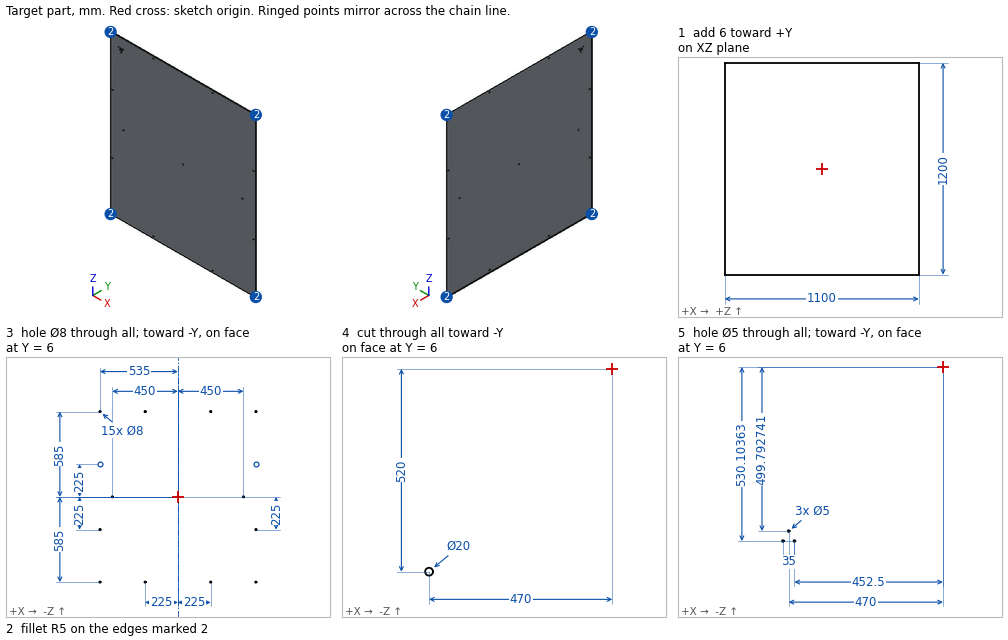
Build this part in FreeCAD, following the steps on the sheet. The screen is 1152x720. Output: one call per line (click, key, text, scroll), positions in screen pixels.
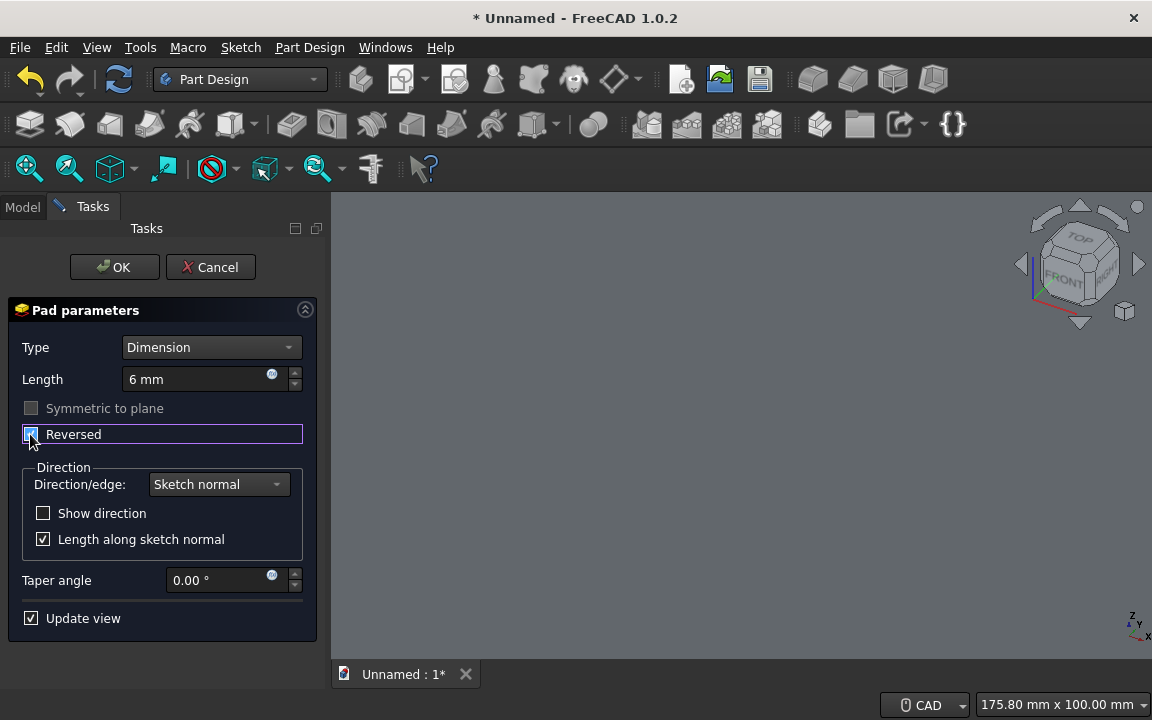
click(115, 267)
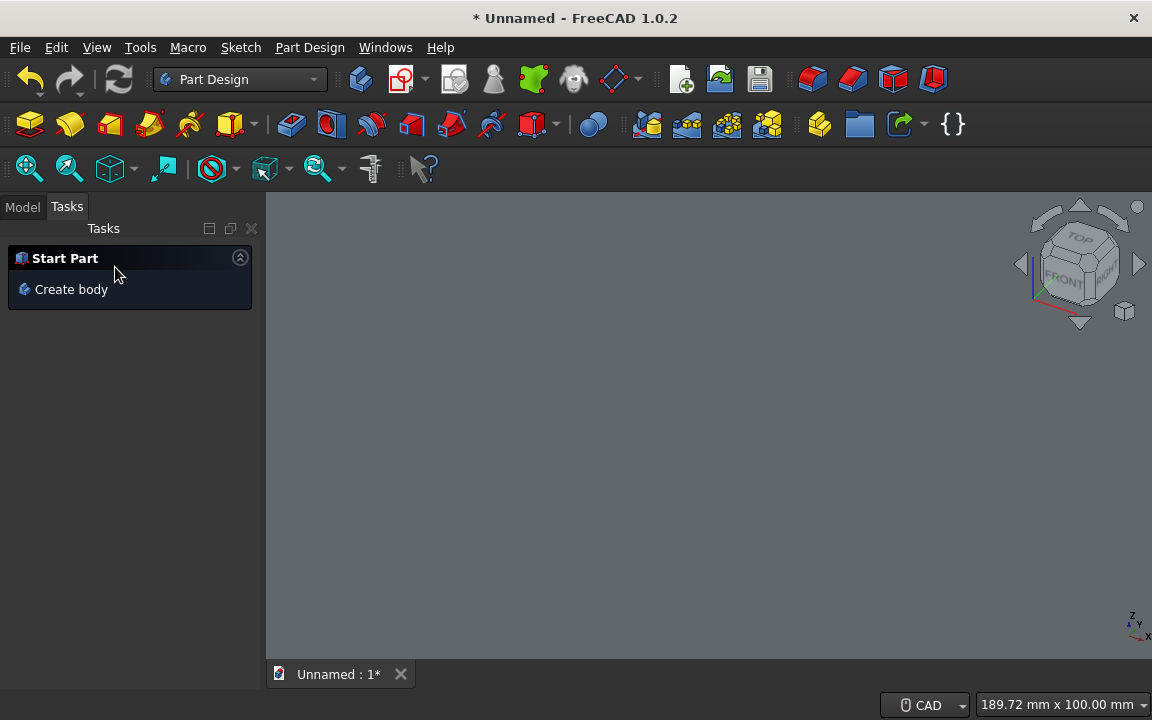
click(30, 170)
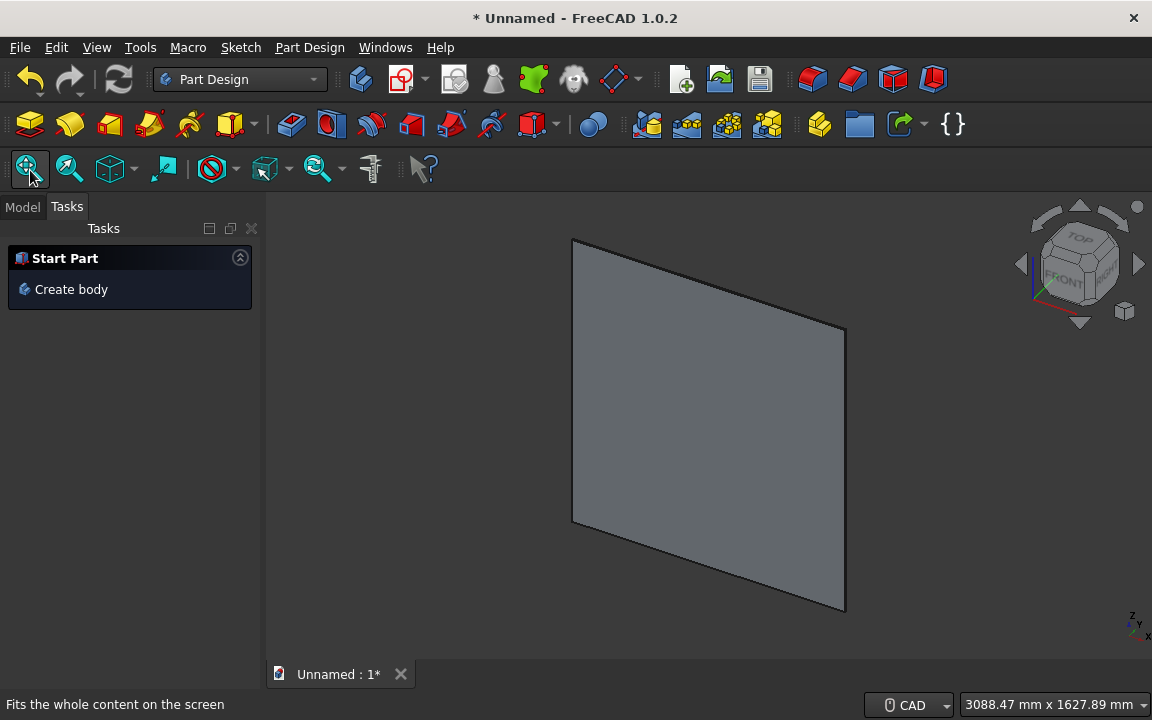
scroll(846, 329, up, 15)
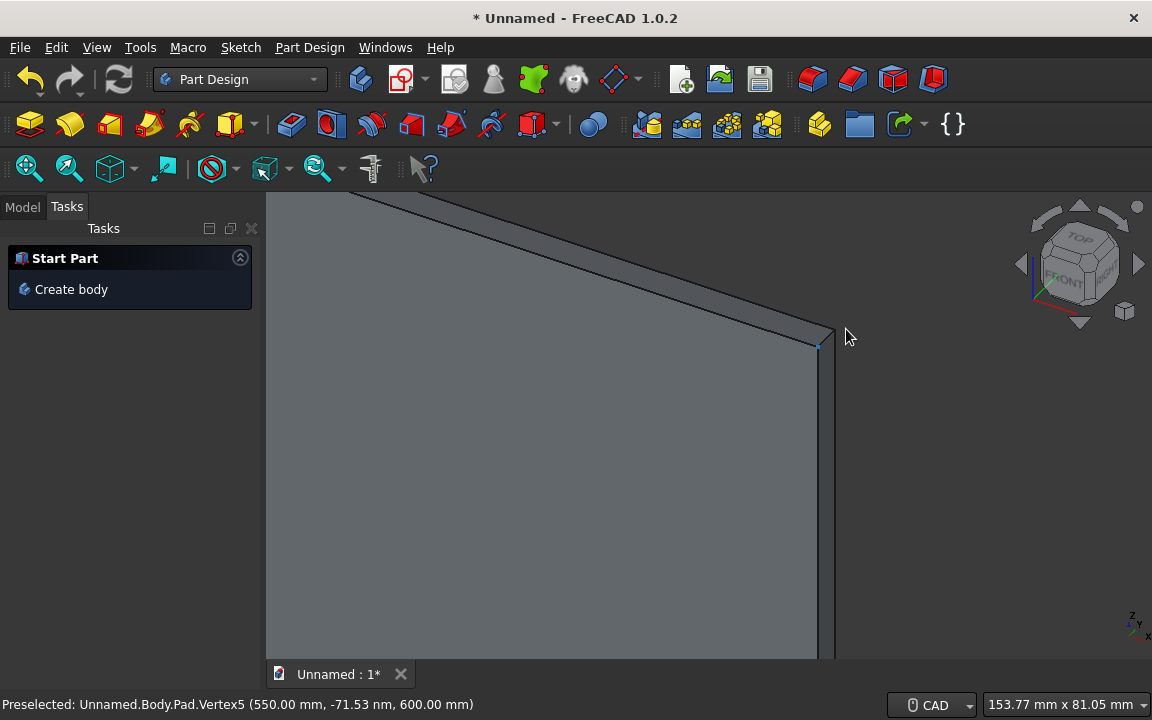
click(826, 338)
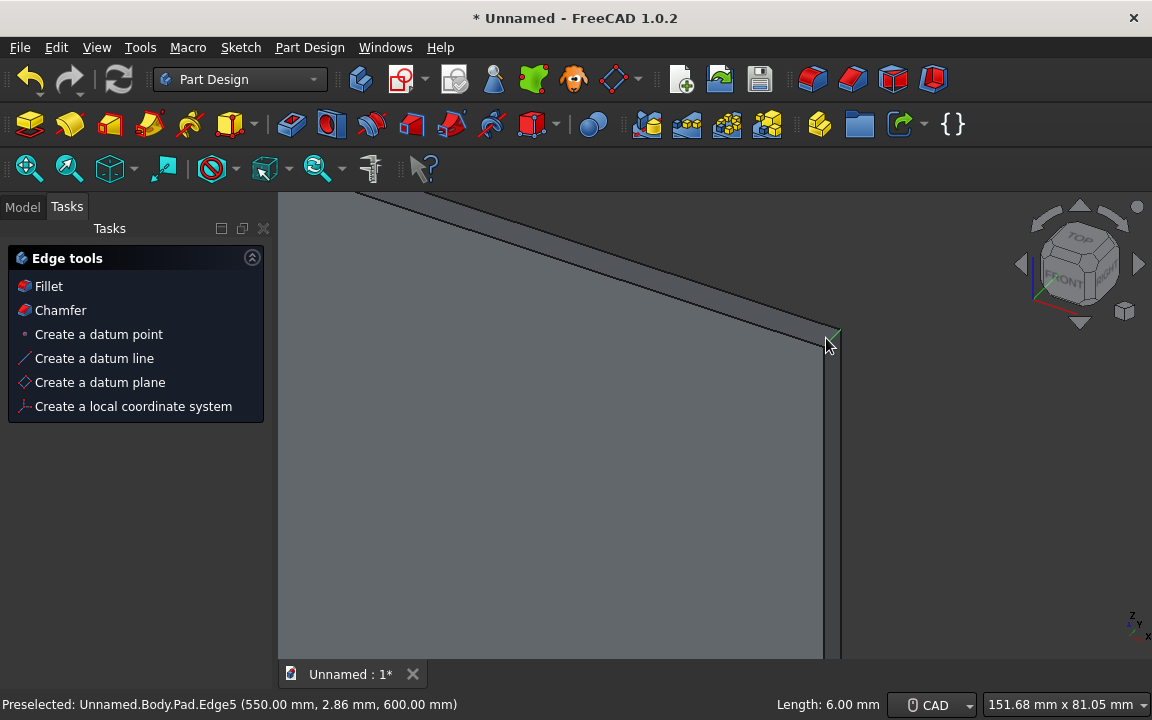
click(30, 170)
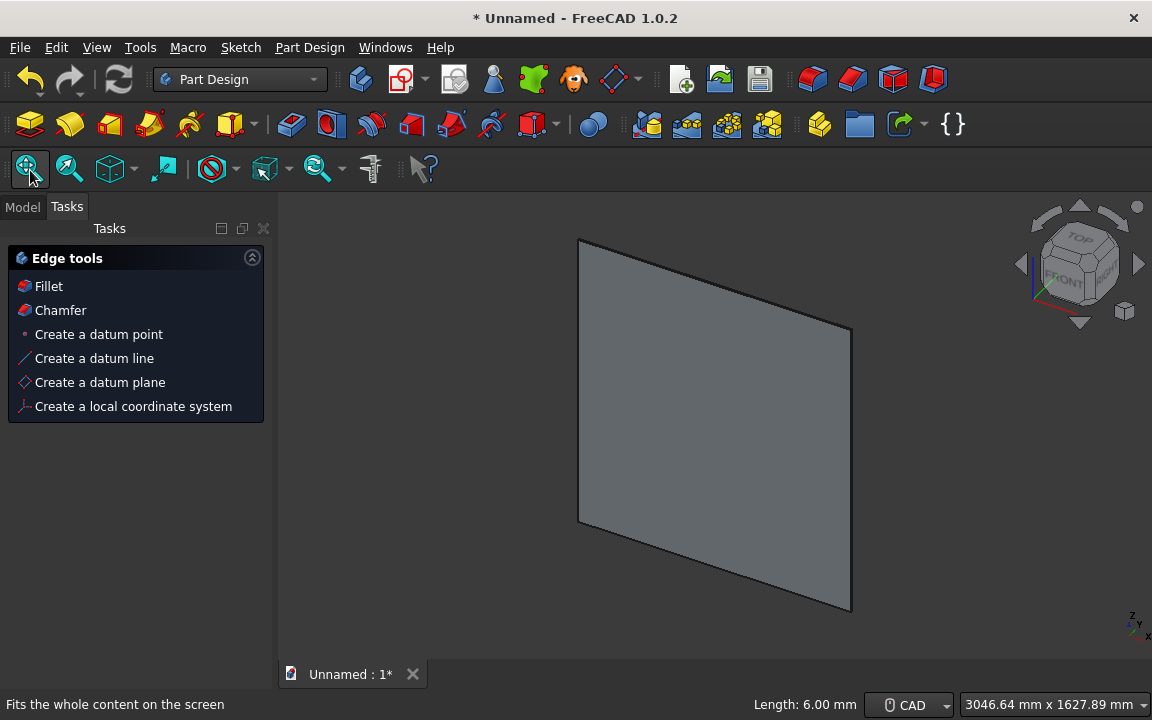
key(0)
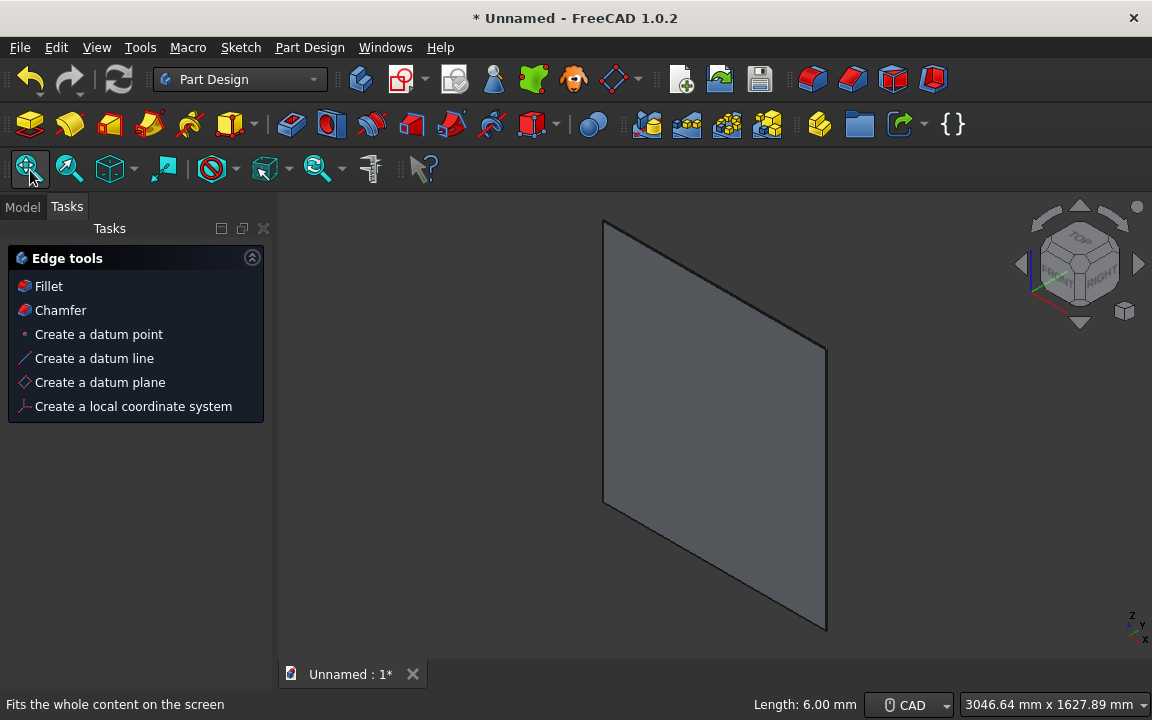
key(2)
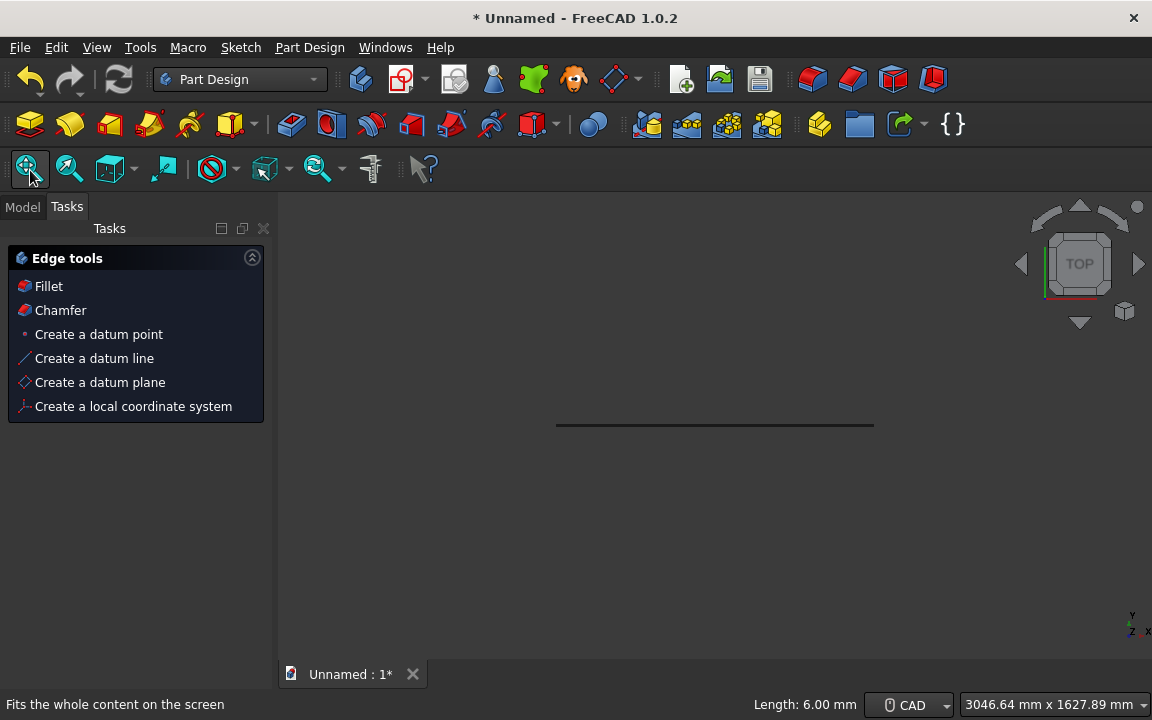
click(30, 170)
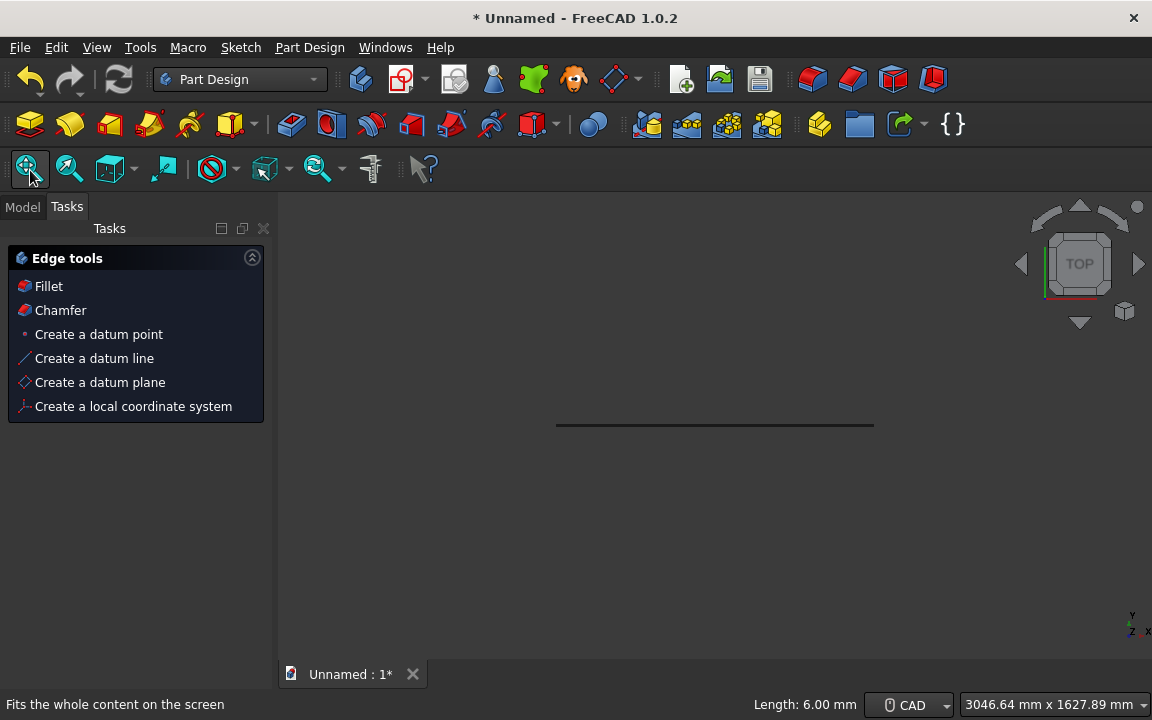
scroll(557, 424, up, 15)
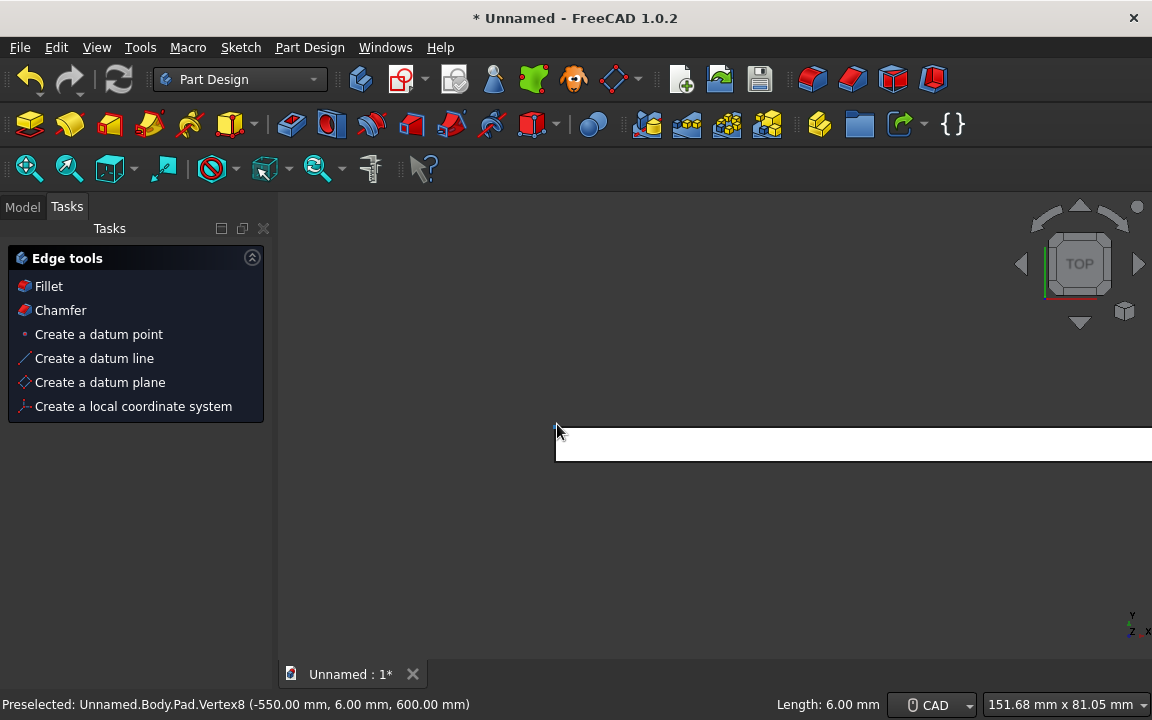
click(555, 444, ctrl)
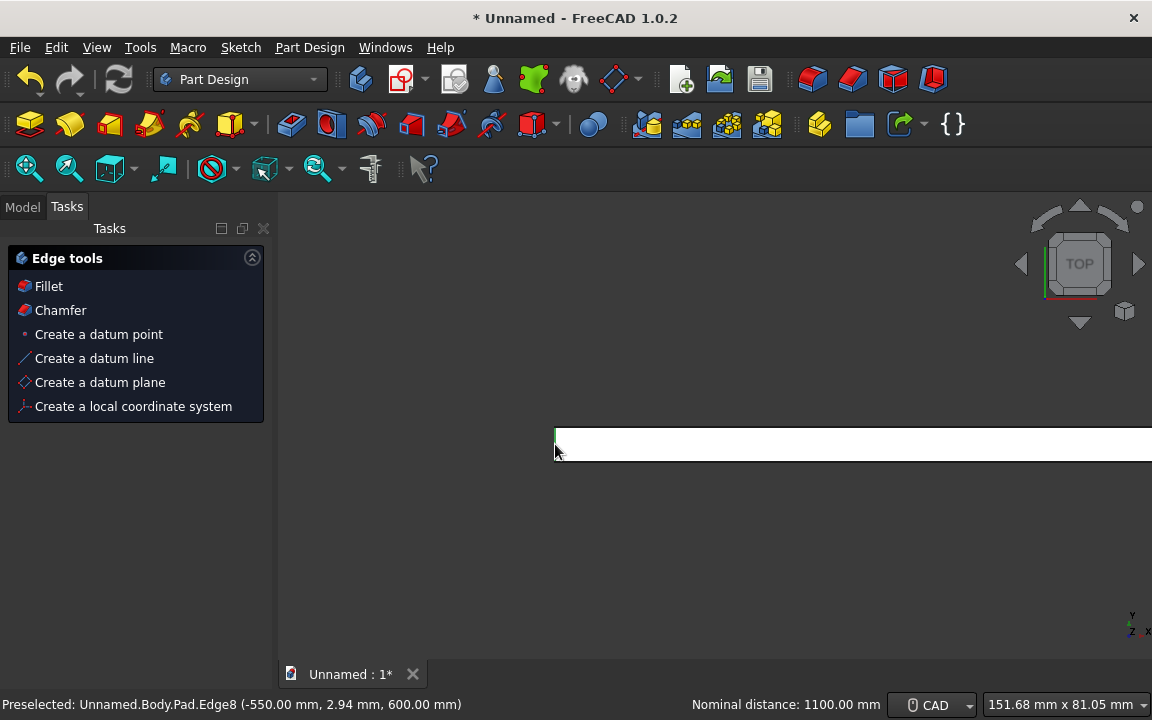
click(30, 170)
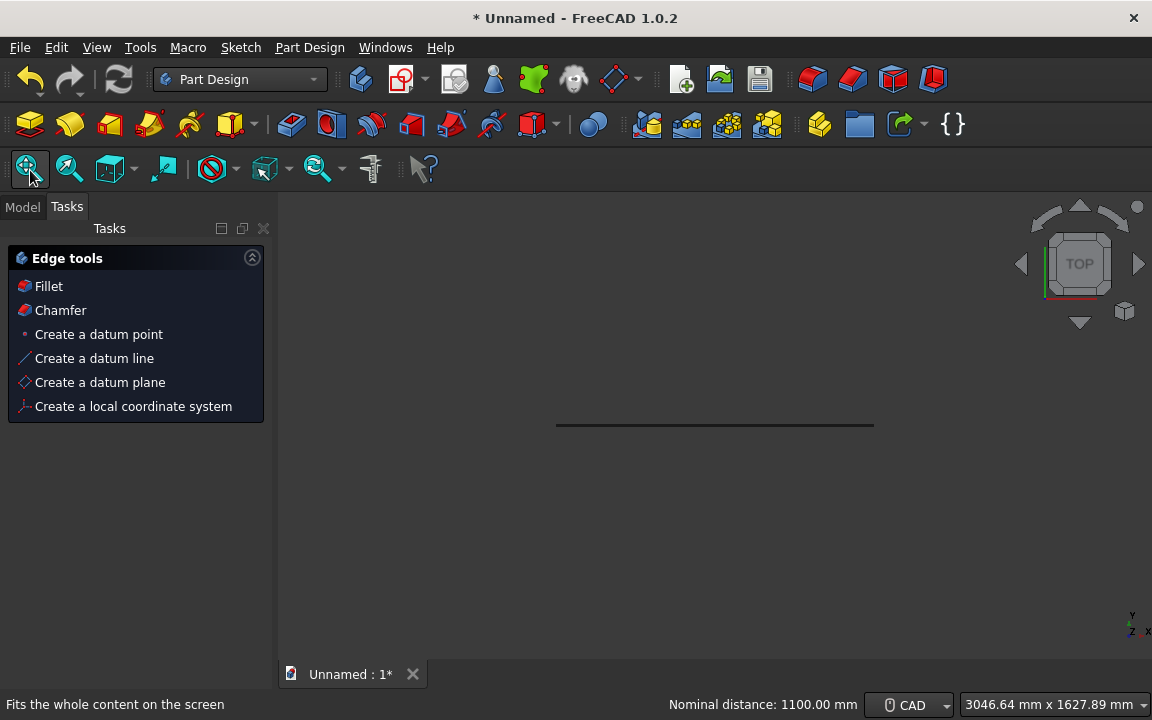
key(1)